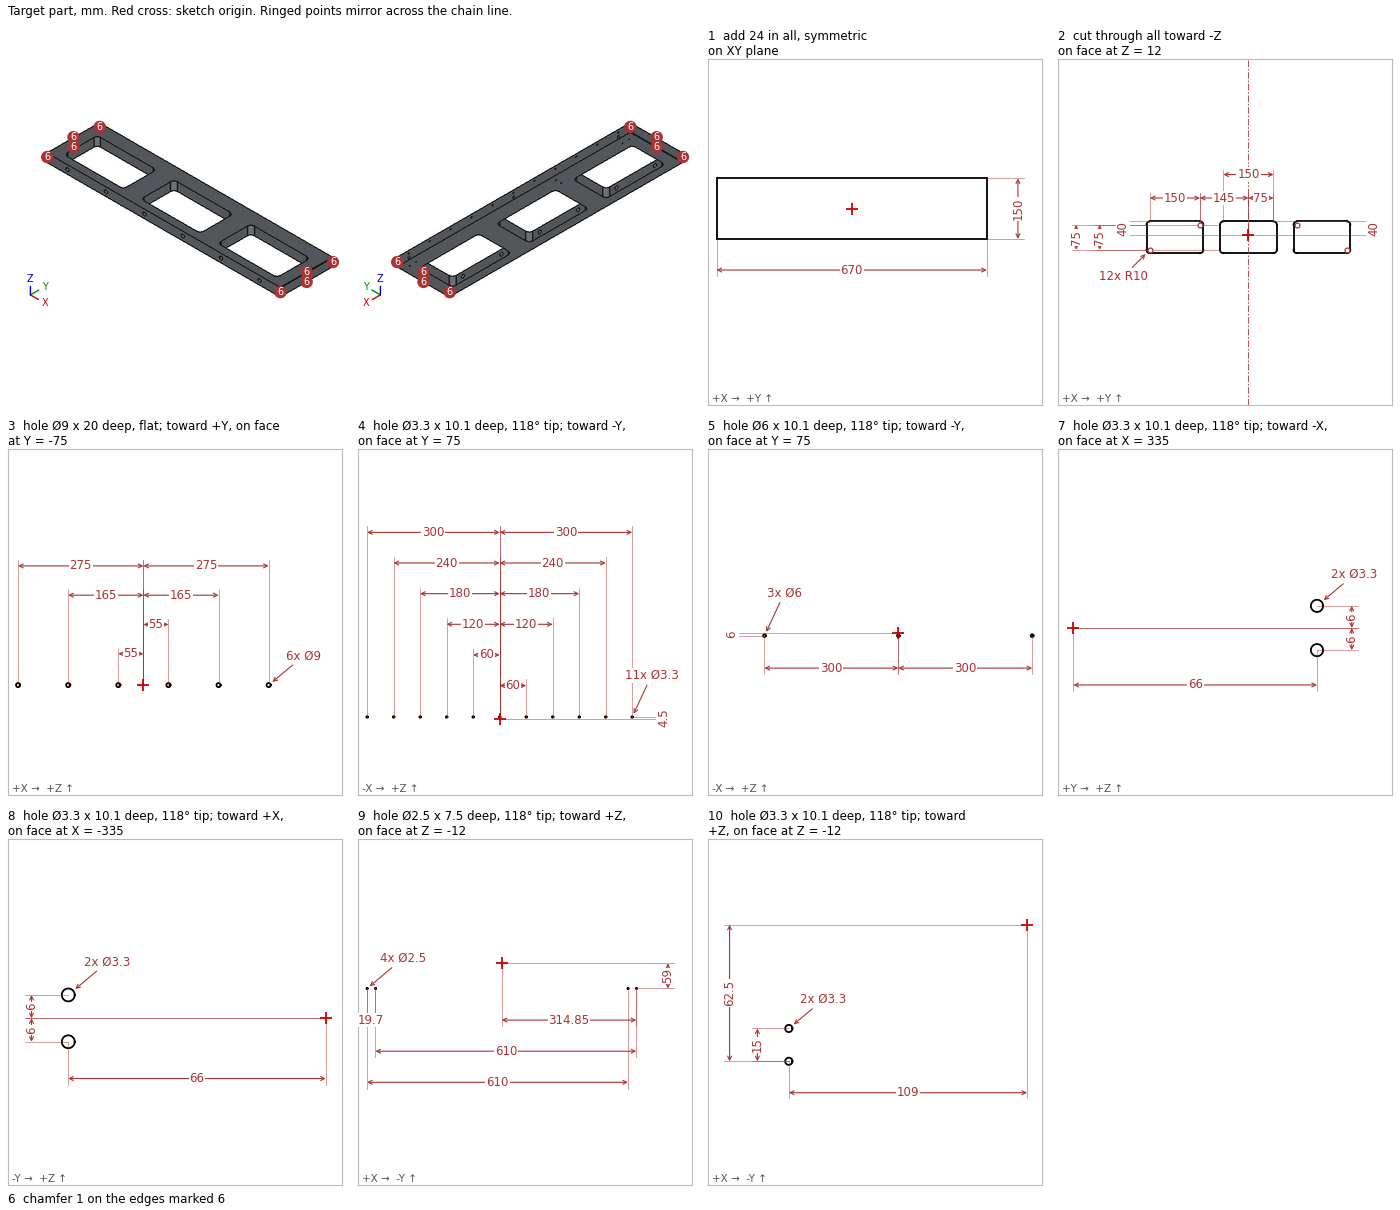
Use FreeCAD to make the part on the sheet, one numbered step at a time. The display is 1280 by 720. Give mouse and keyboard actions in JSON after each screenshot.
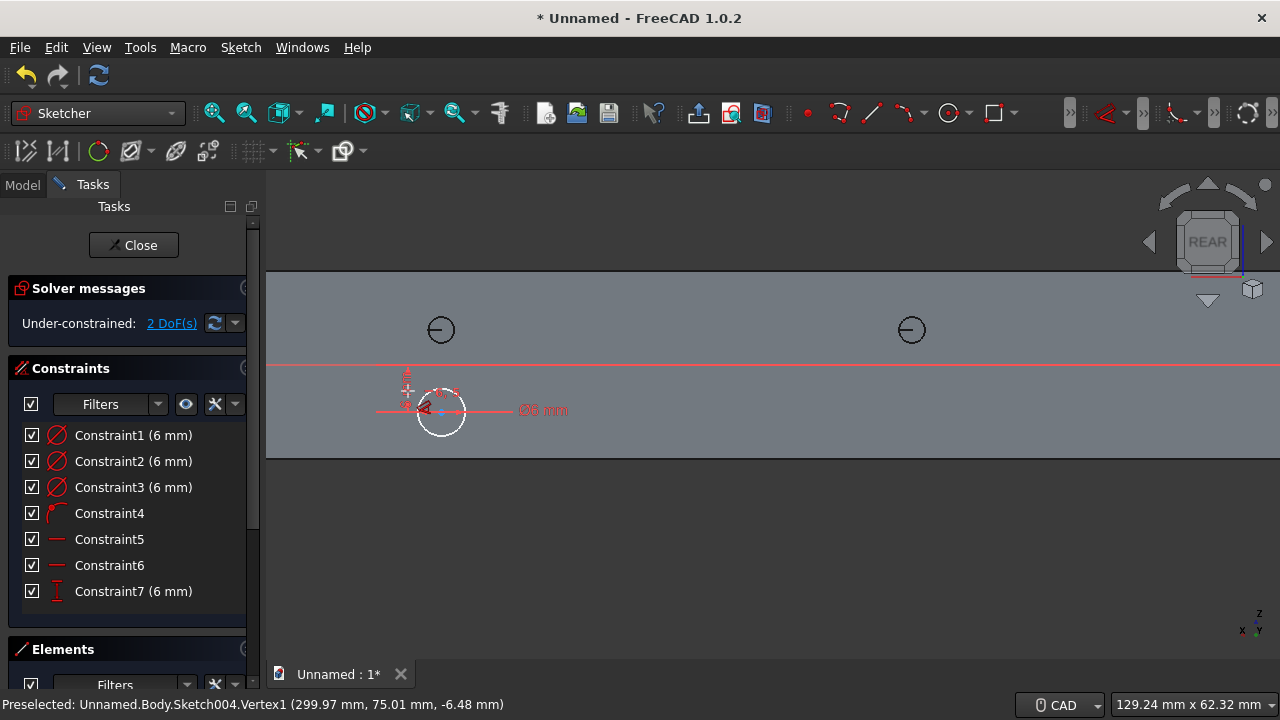
{"action": "scroll", "coordinate": [444, 416], "scroll_direction": "down", "scroll_amount": 11}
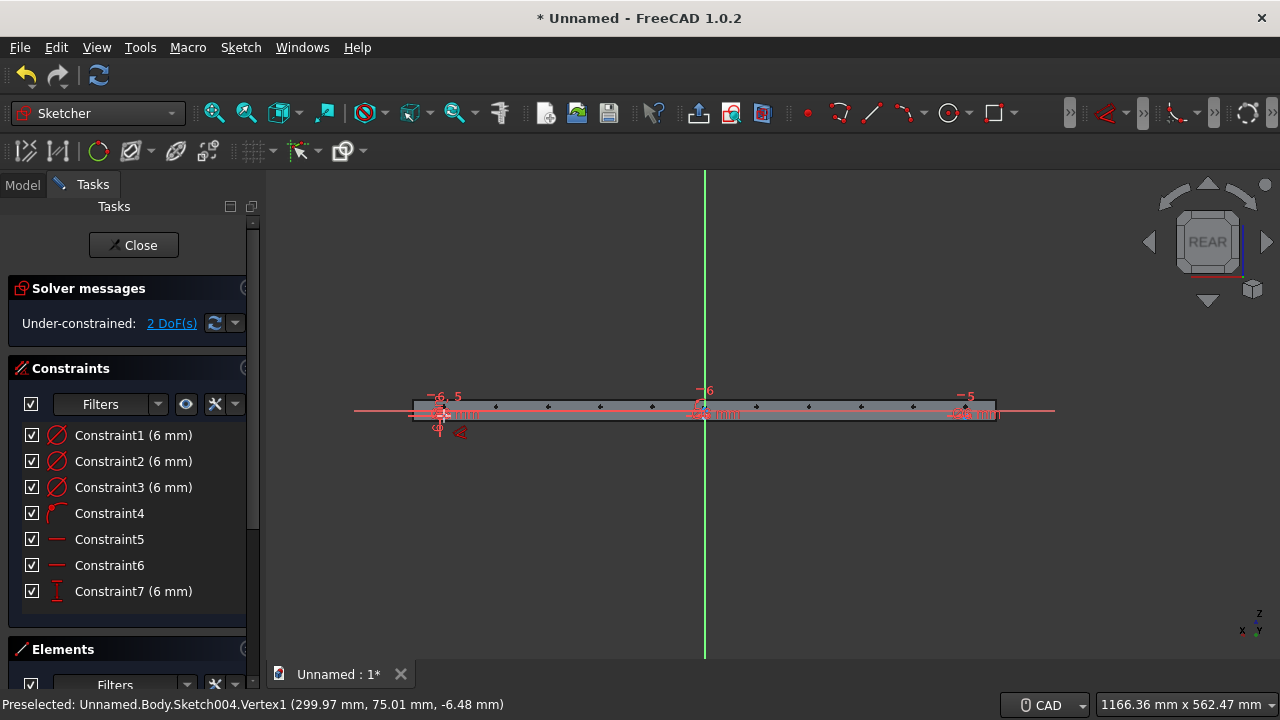
{"action": "left_click", "coordinate": [444, 416]}
{"action": "left_click", "coordinate": [574, 377]}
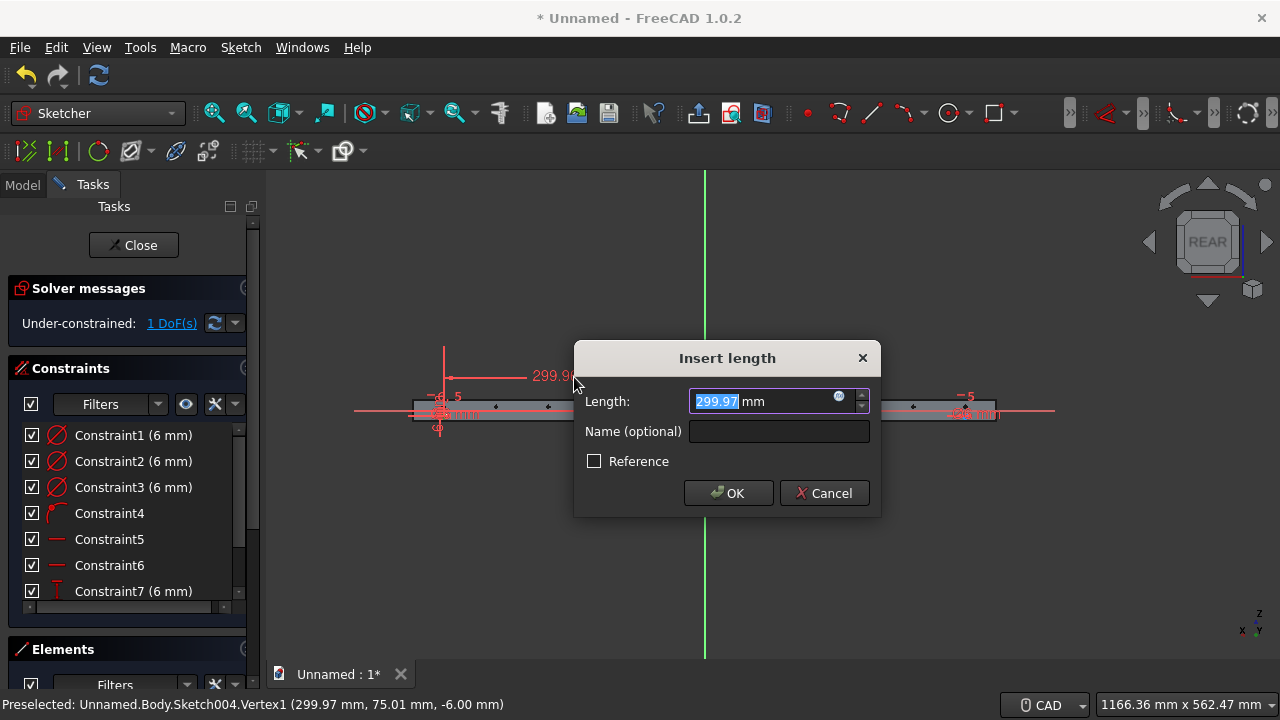
{"action": "type", "text": "300"}
{"action": "key", "text": "Return"}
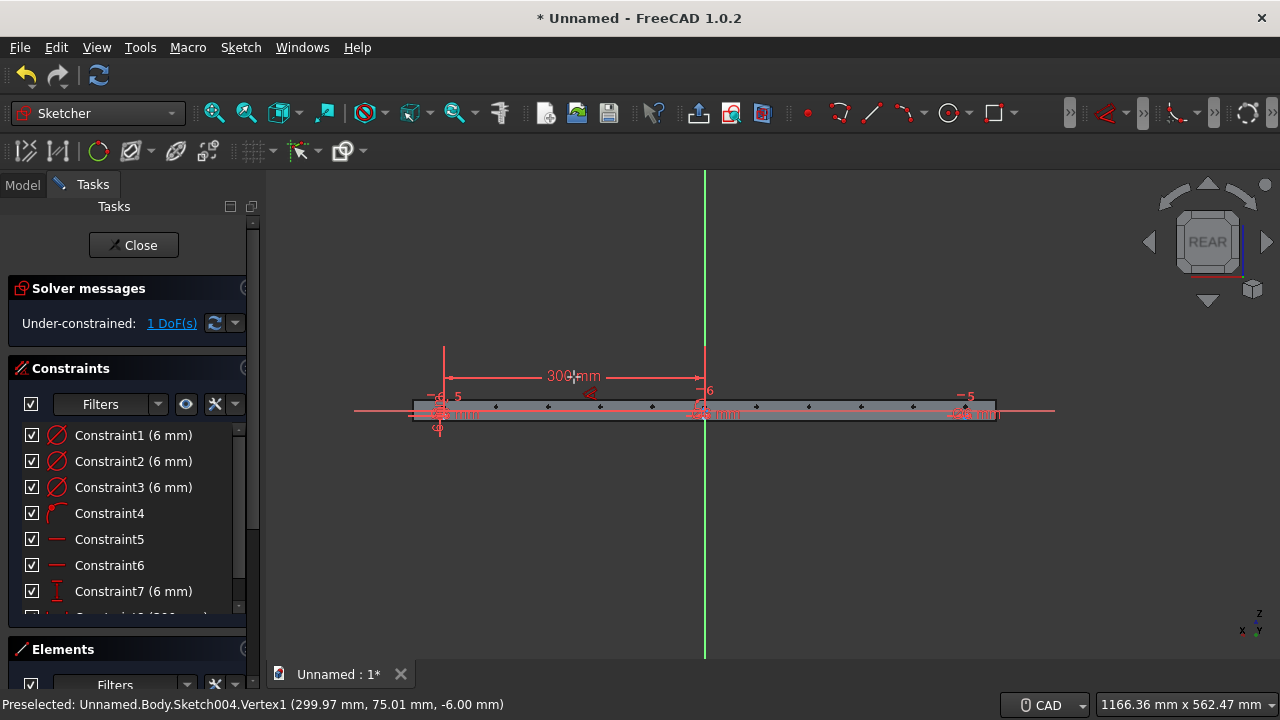
{"action": "left_click", "coordinate": [965, 416]}
{"action": "left_click", "coordinate": [835, 377]}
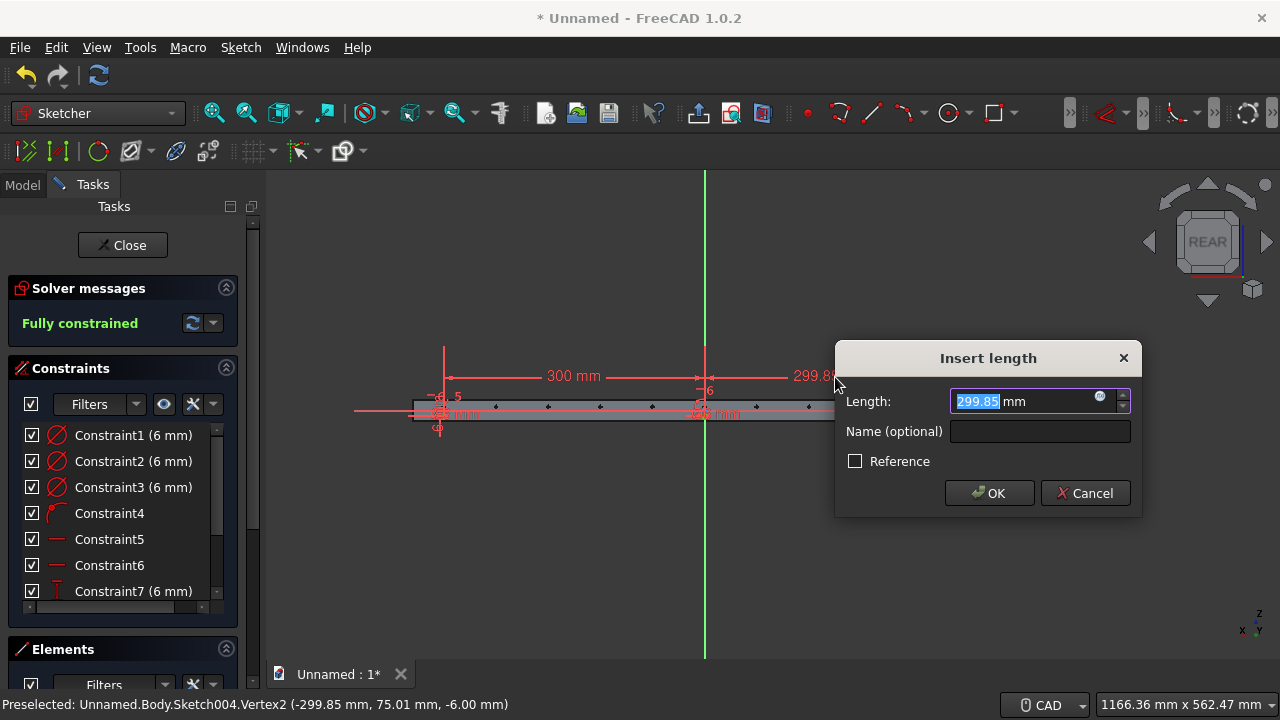
{"action": "type", "text": "300"}
{"action": "key", "text": "Return"}
{"action": "key", "text": "Escape"}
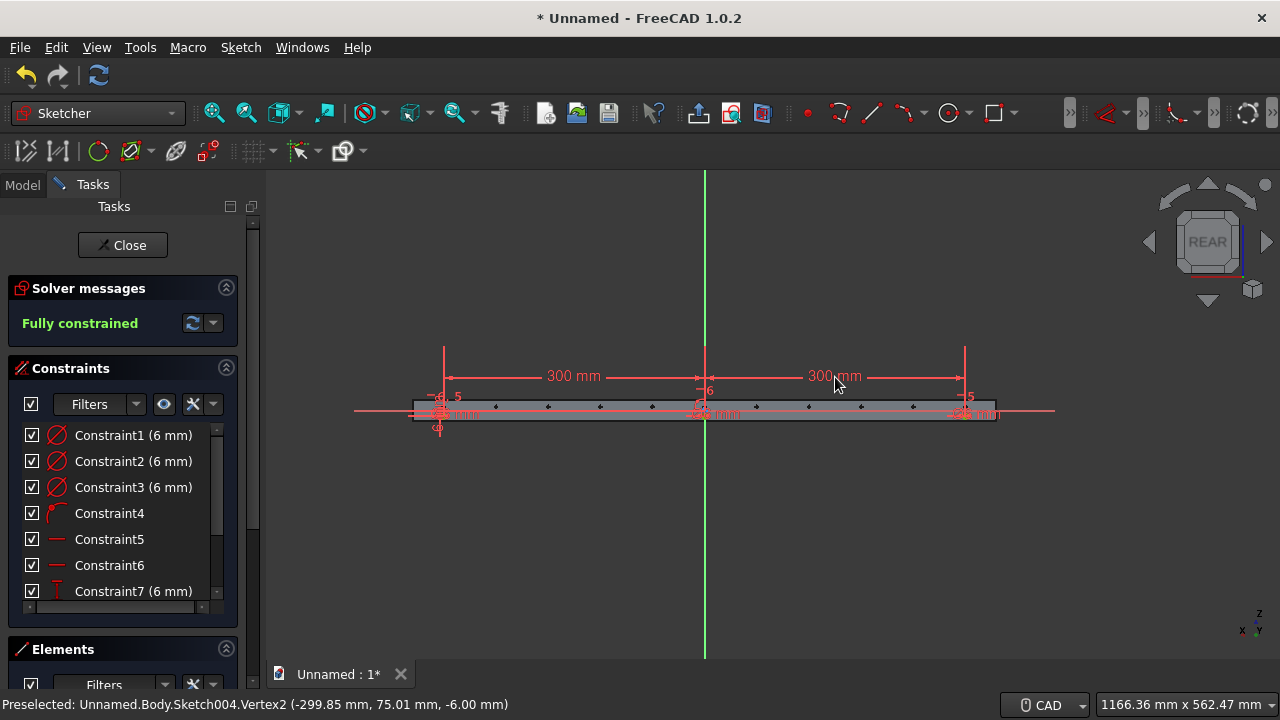
{"action": "left_click", "coordinate": [123, 245]}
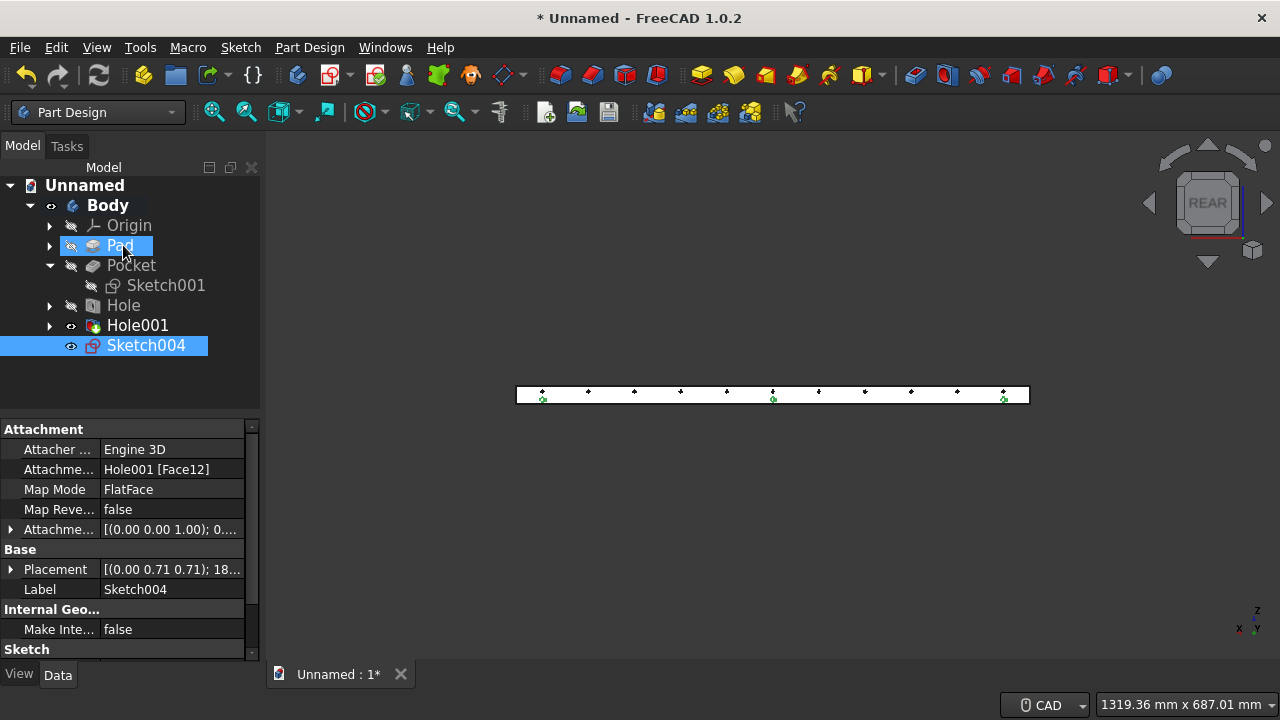
{"action": "left_click", "coordinate": [948, 76]}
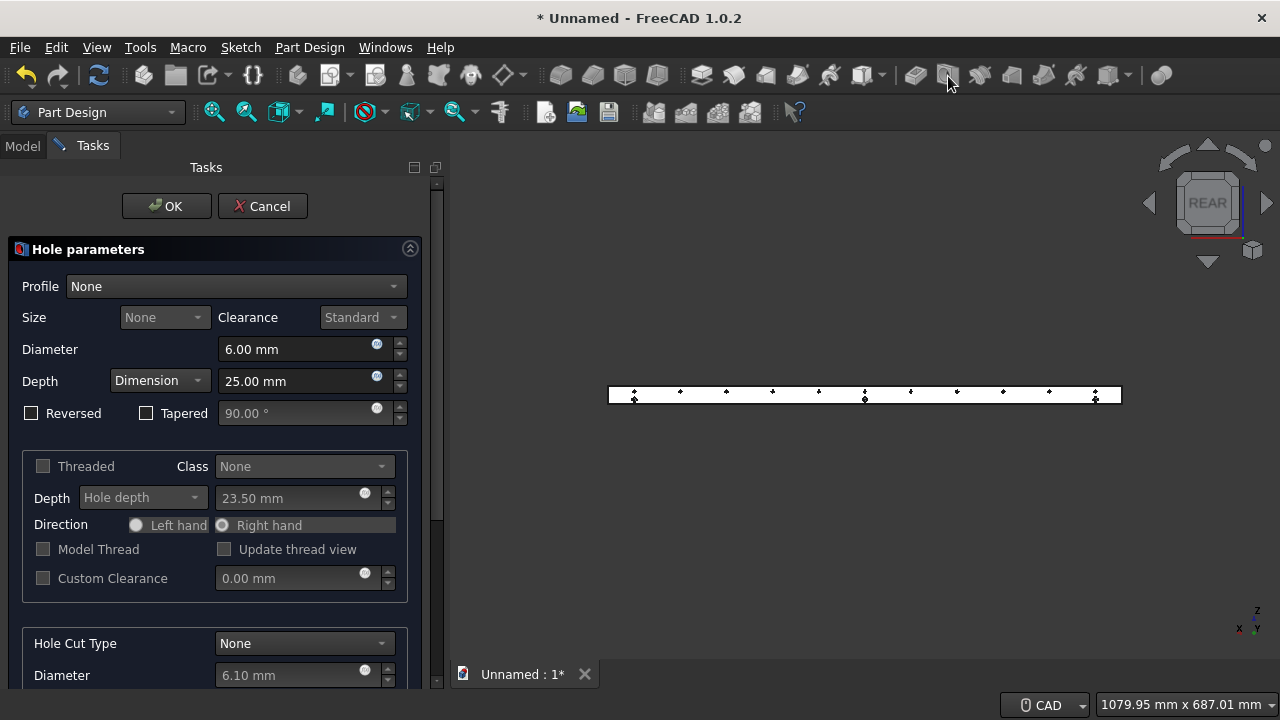
{"action": "triple_click", "coordinate": [305, 349]}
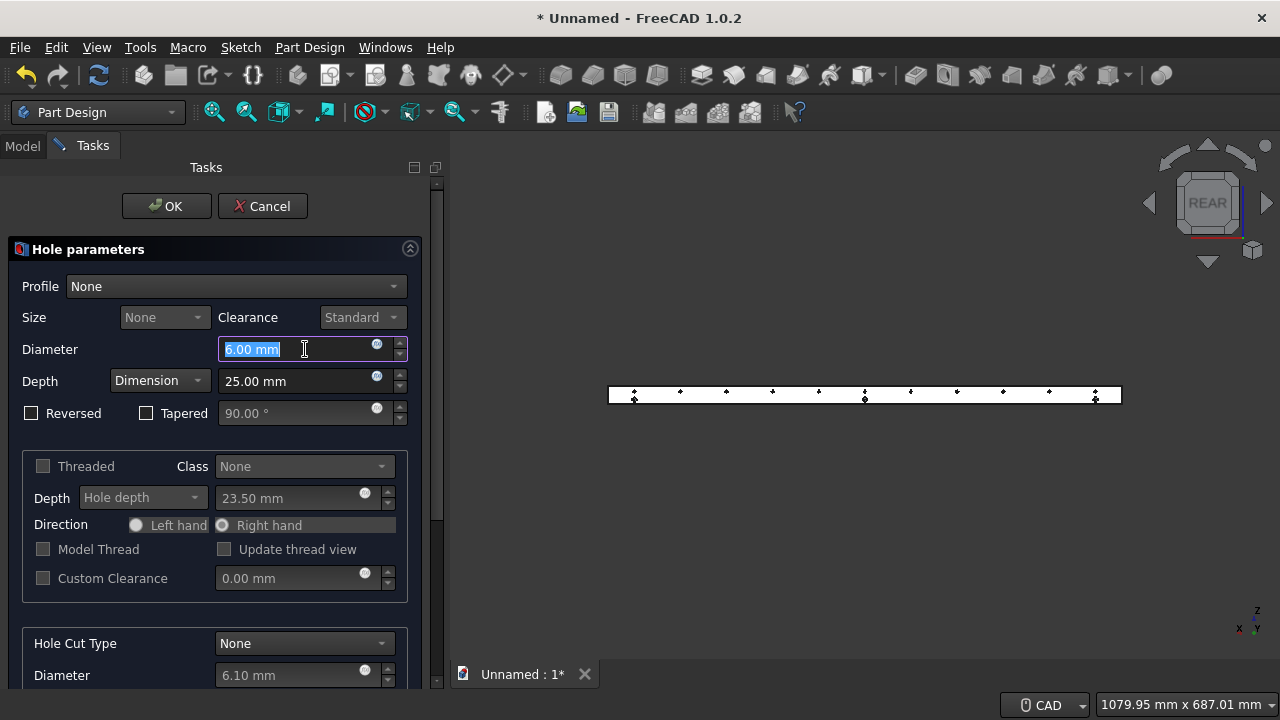
{"action": "type", "text": "6"}
{"action": "key", "text": "Tab"}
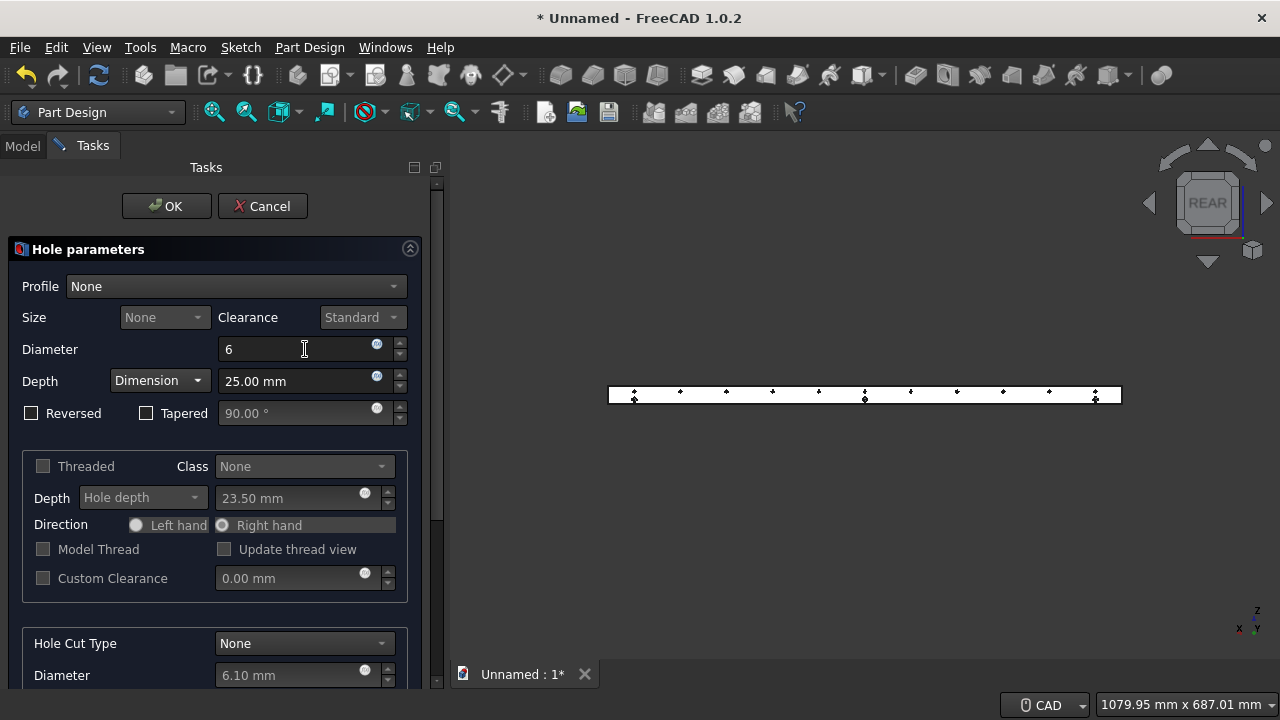
{"action": "triple_click", "coordinate": [305, 381]}